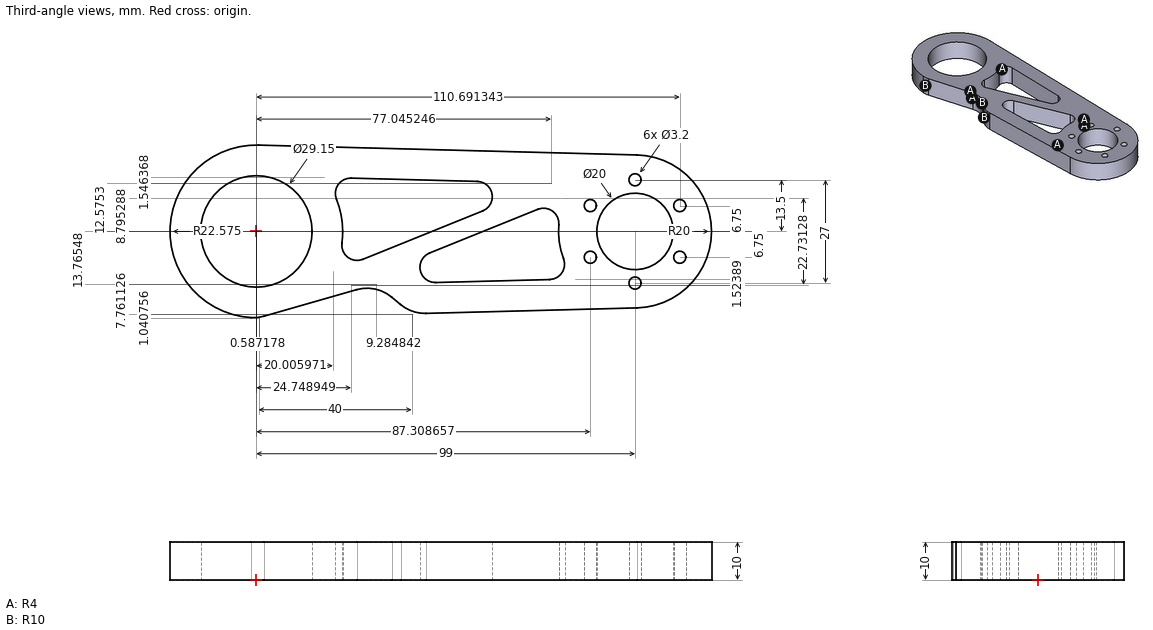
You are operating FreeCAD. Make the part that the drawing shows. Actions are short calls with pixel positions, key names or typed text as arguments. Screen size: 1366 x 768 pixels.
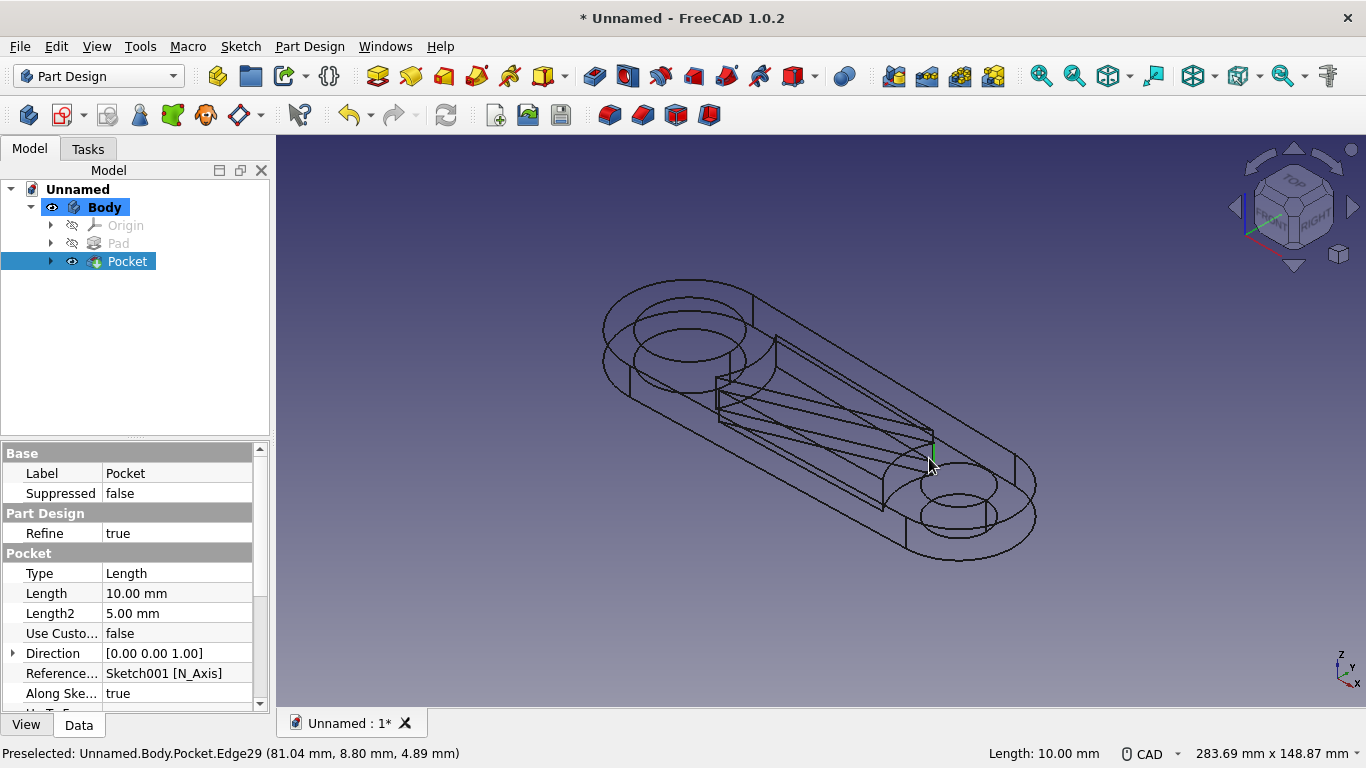
click(883, 494, ctrl)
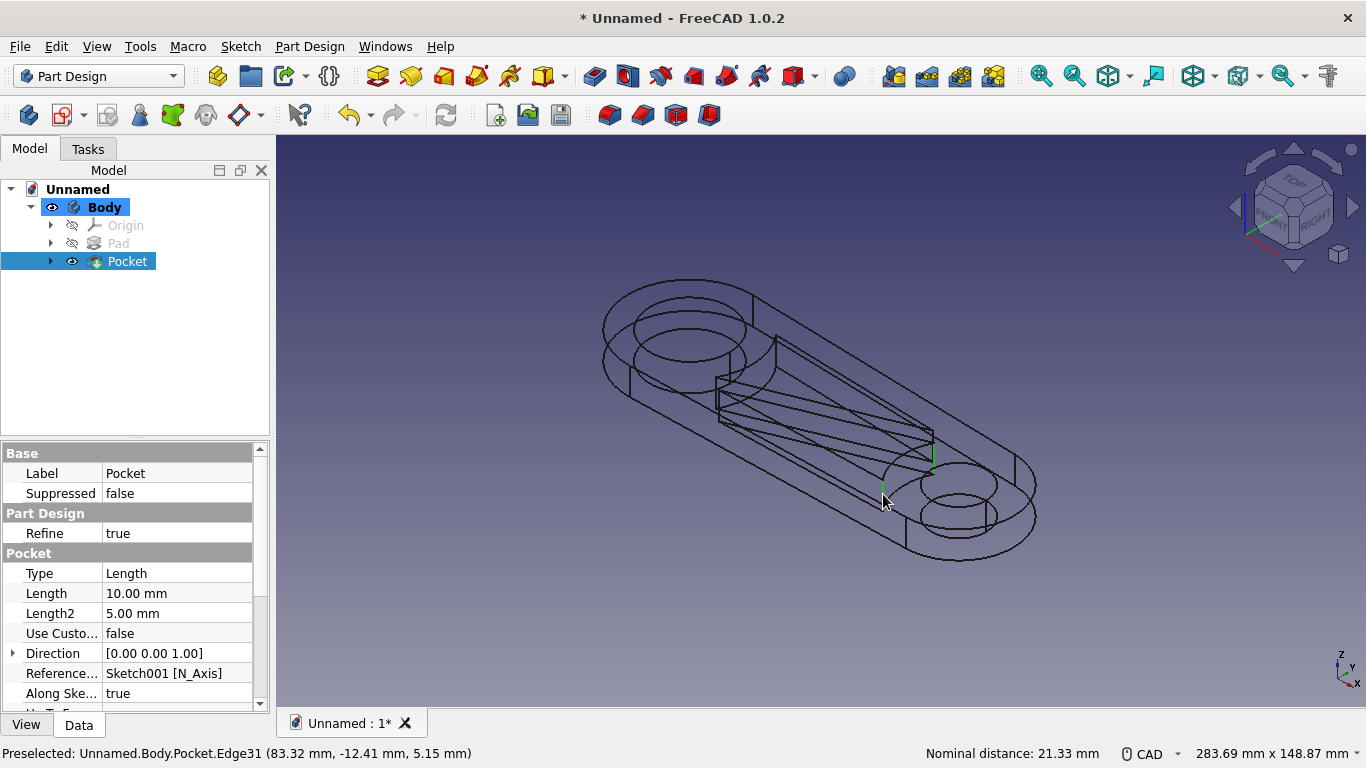
click(719, 405, ctrl)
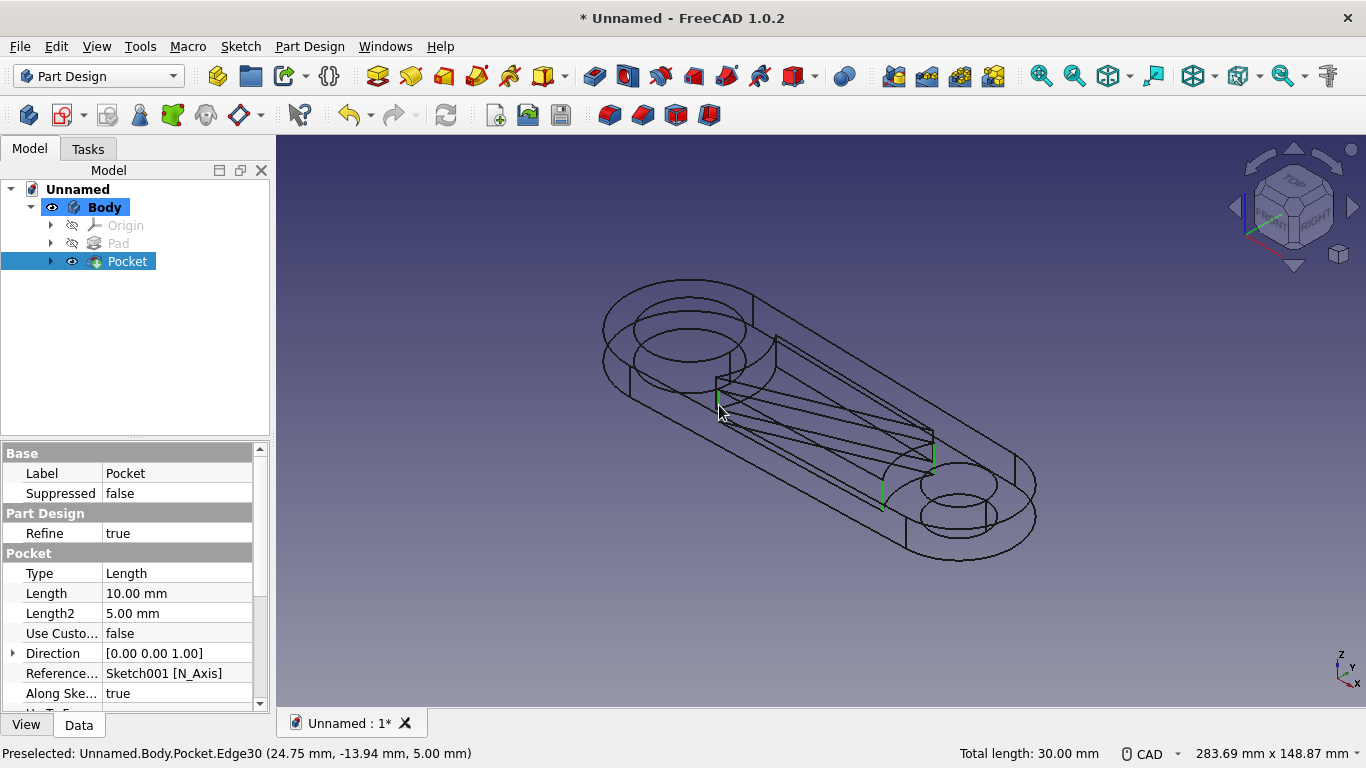
click(716, 383, ctrl)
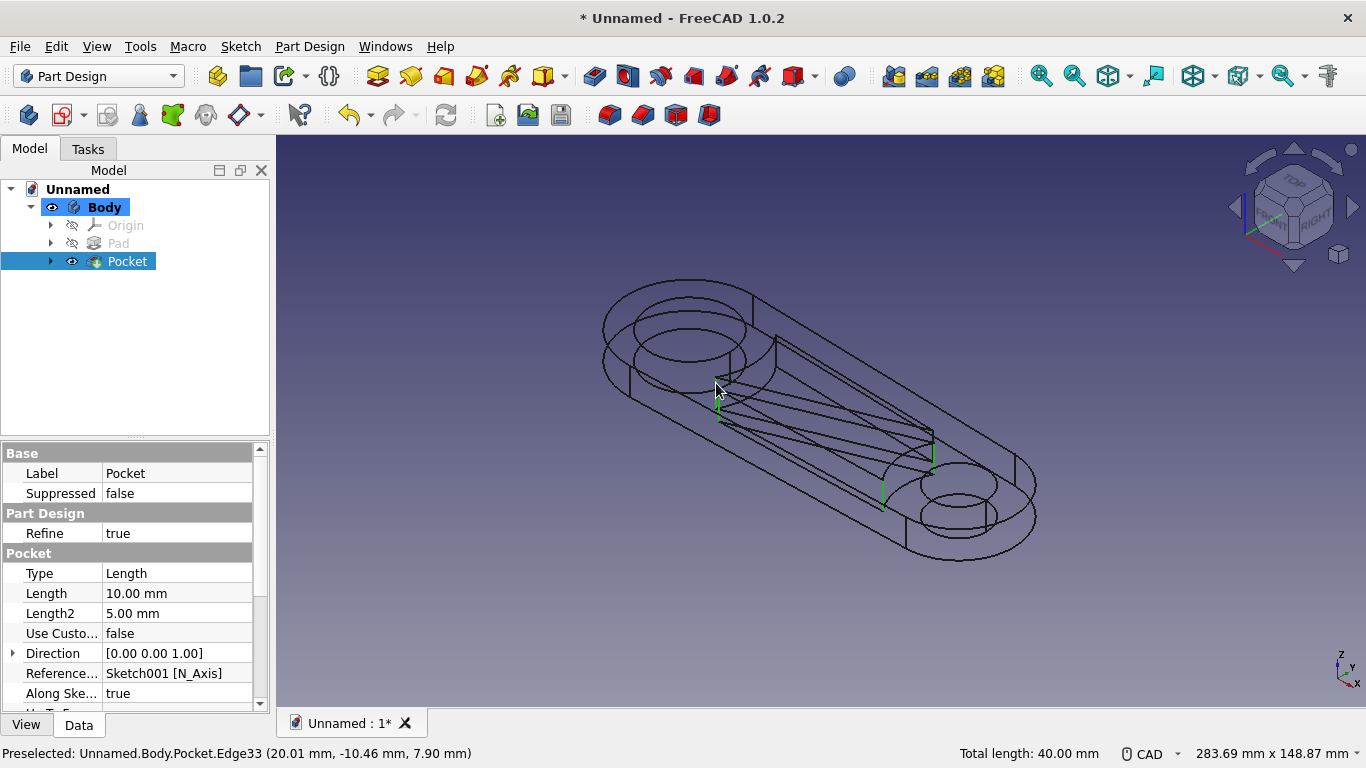
click(776, 353, ctrl)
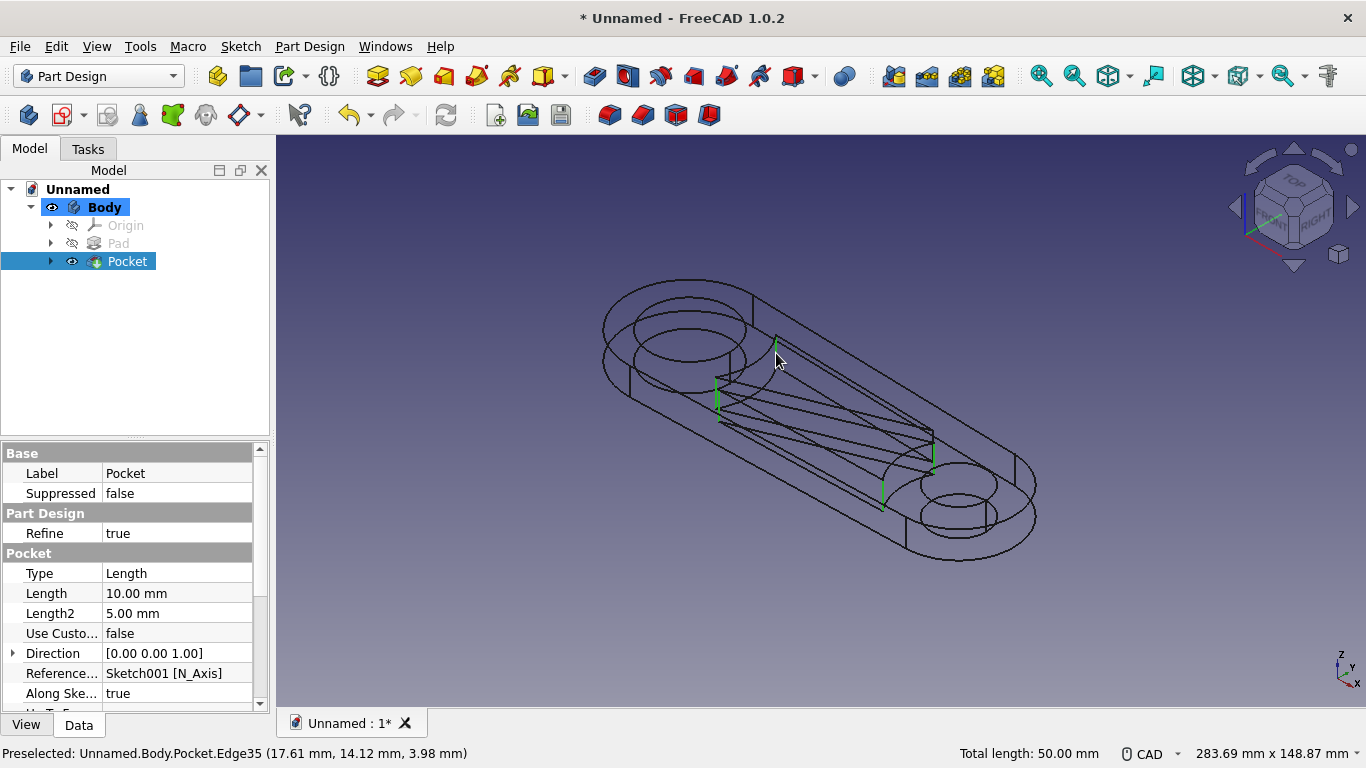
scroll(933, 445, up, 6)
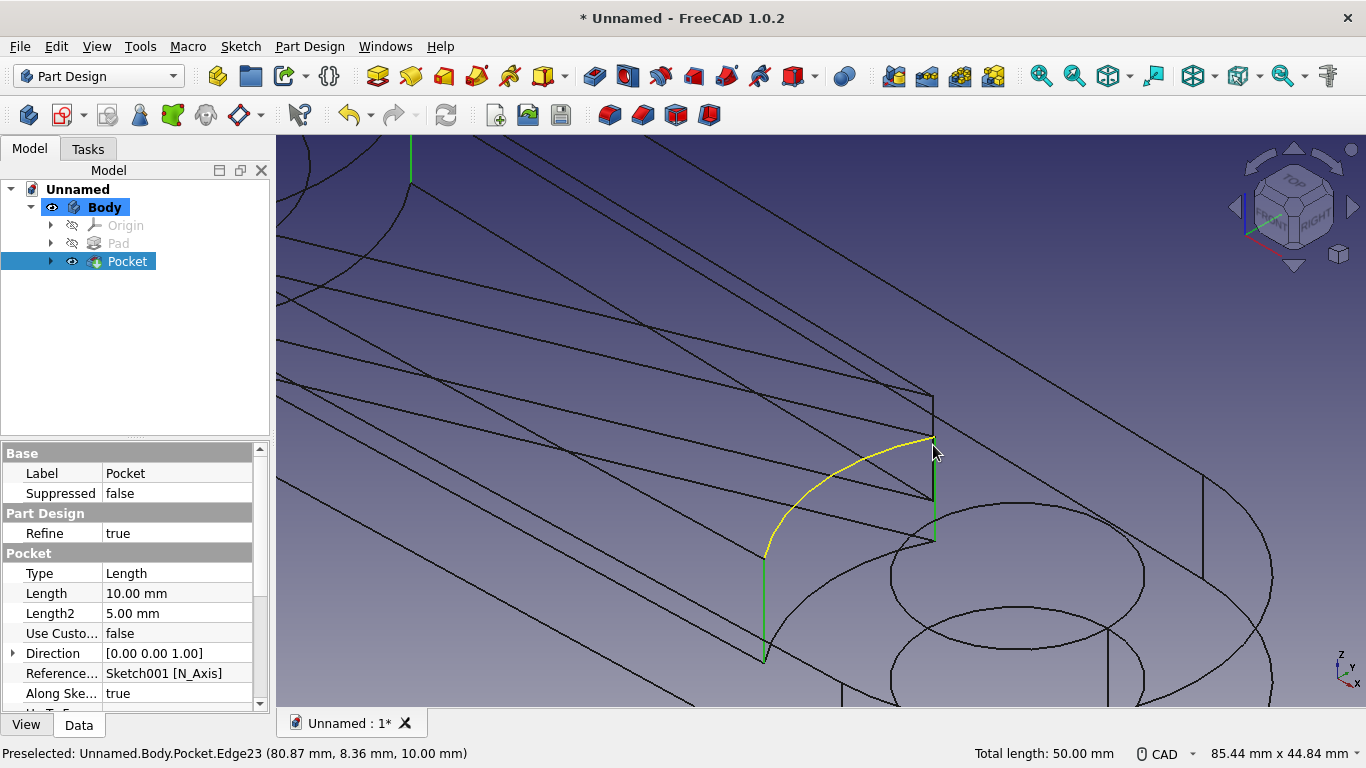
click(933, 427, ctrl)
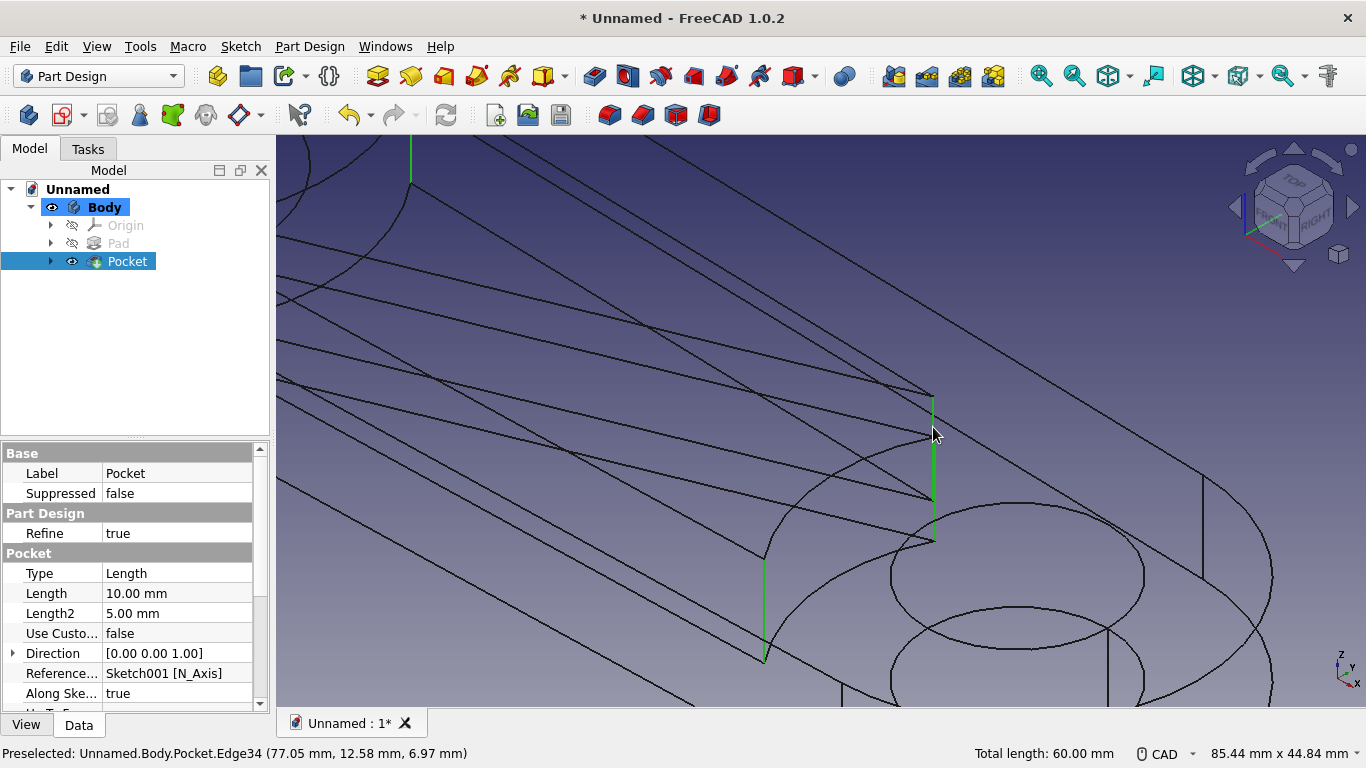
key(v)
key(1)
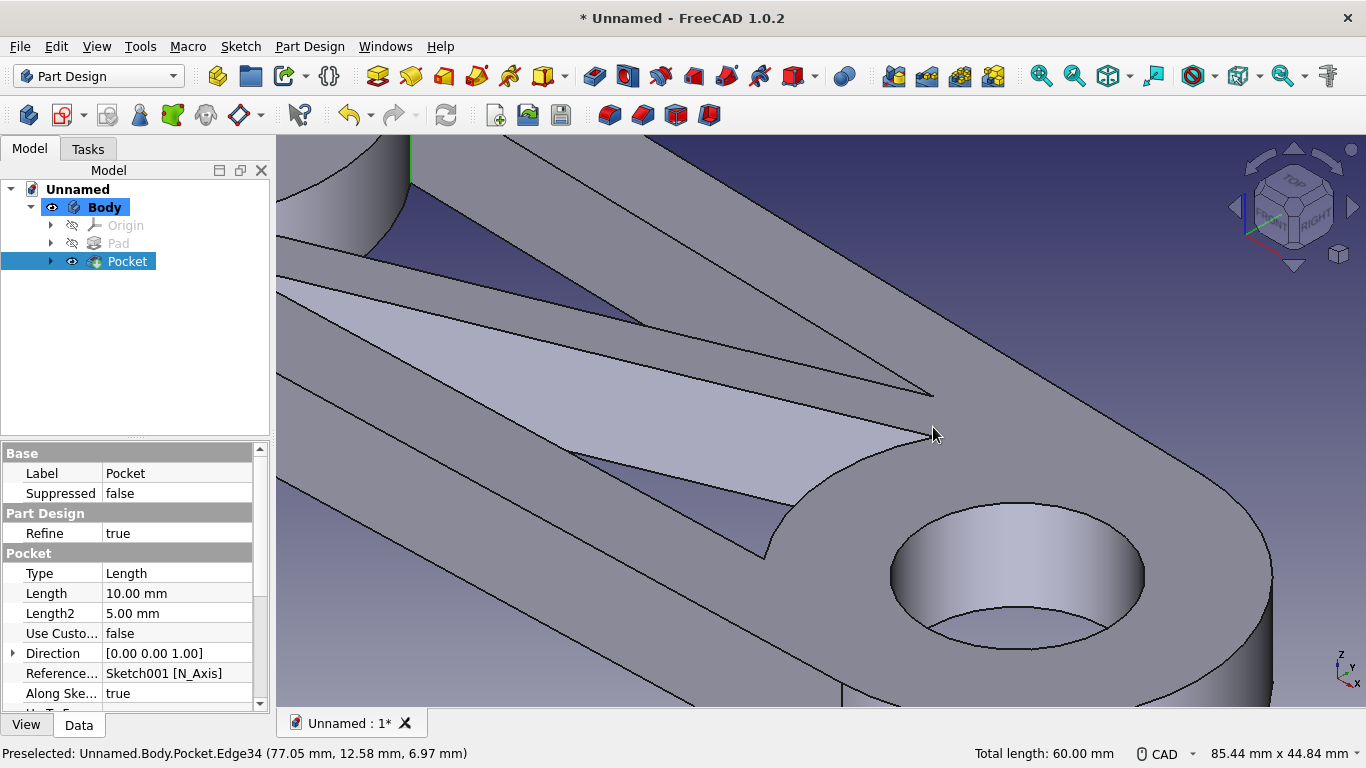
click(610, 116)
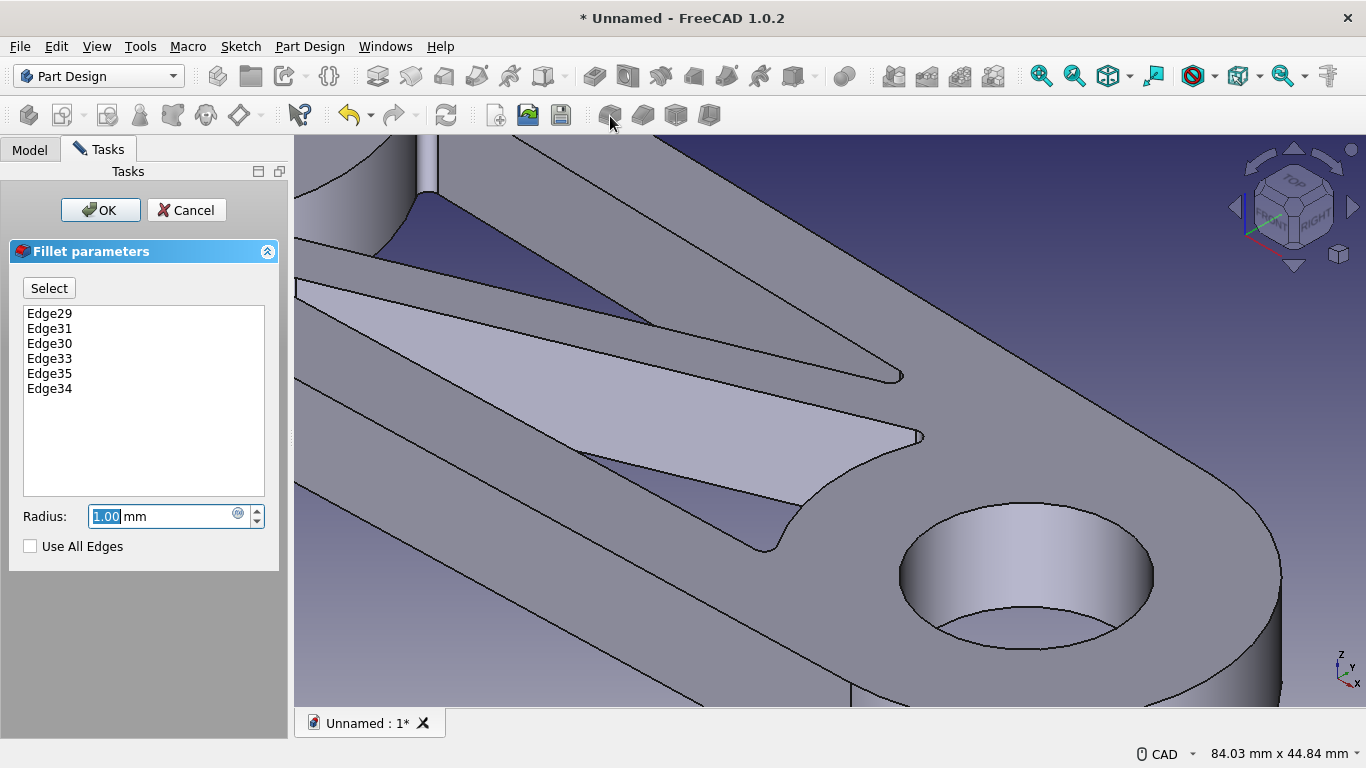
text(4)
key(Tab)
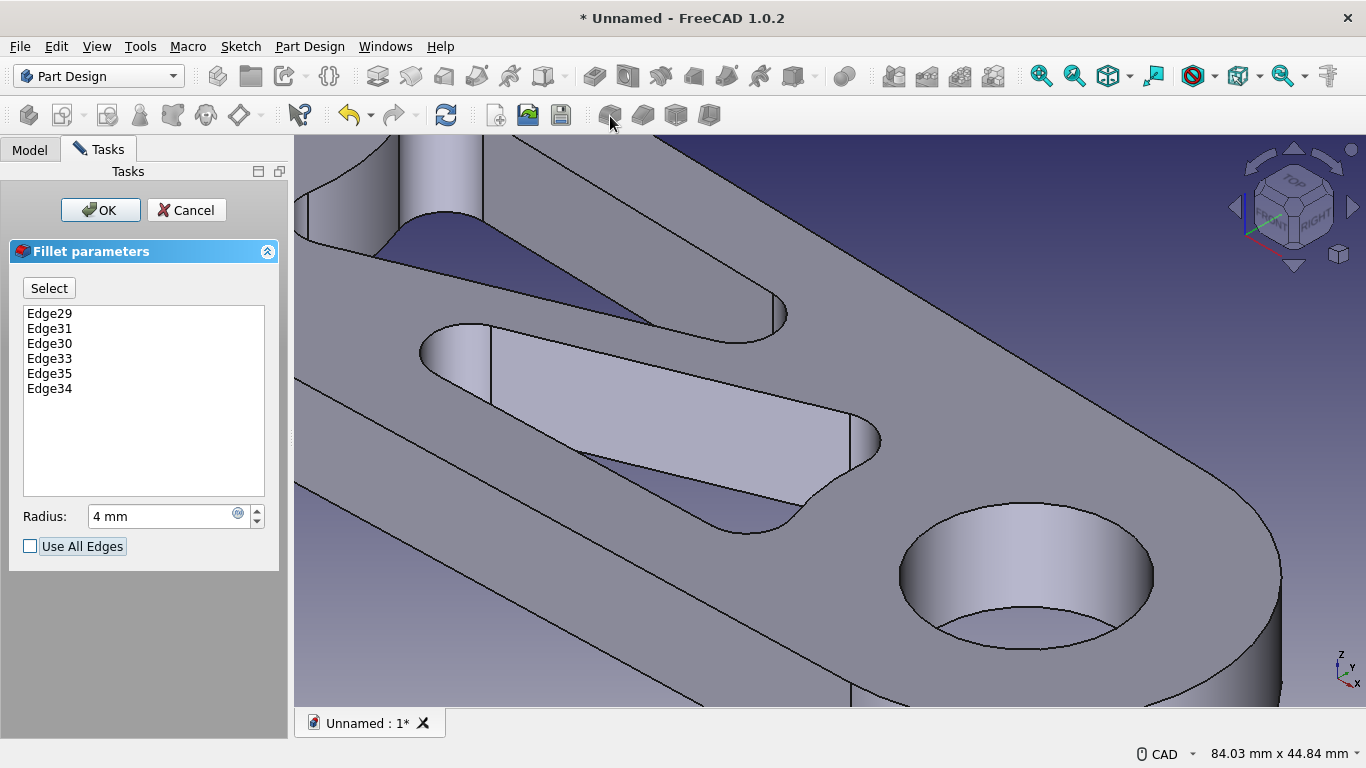
click(101, 210)